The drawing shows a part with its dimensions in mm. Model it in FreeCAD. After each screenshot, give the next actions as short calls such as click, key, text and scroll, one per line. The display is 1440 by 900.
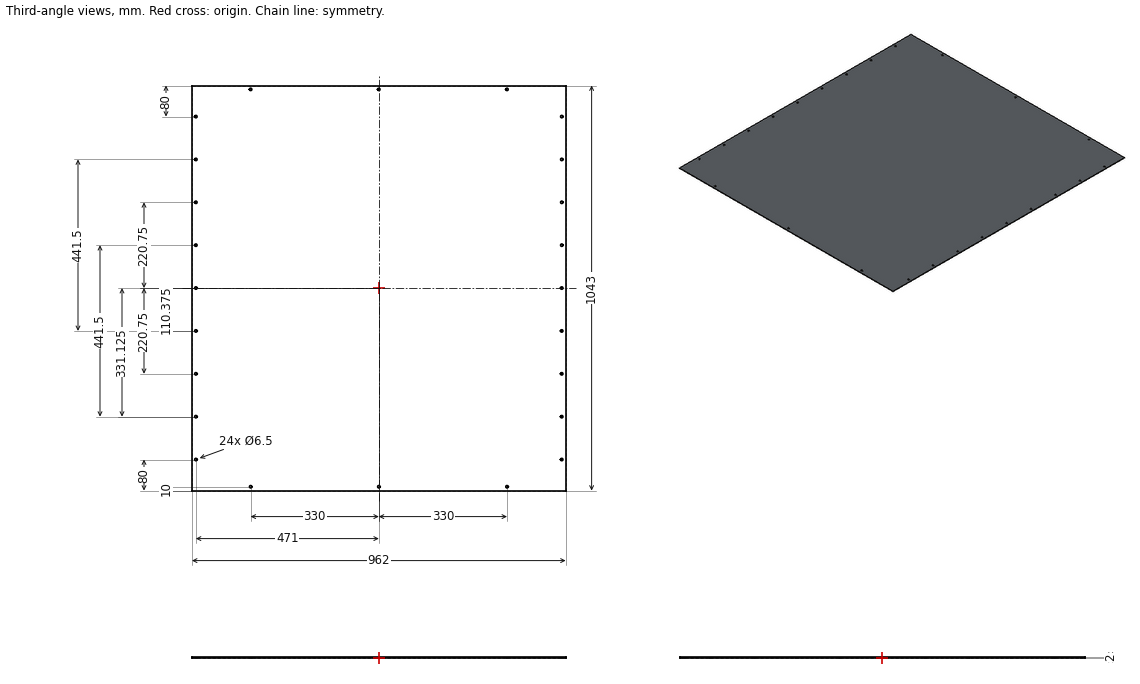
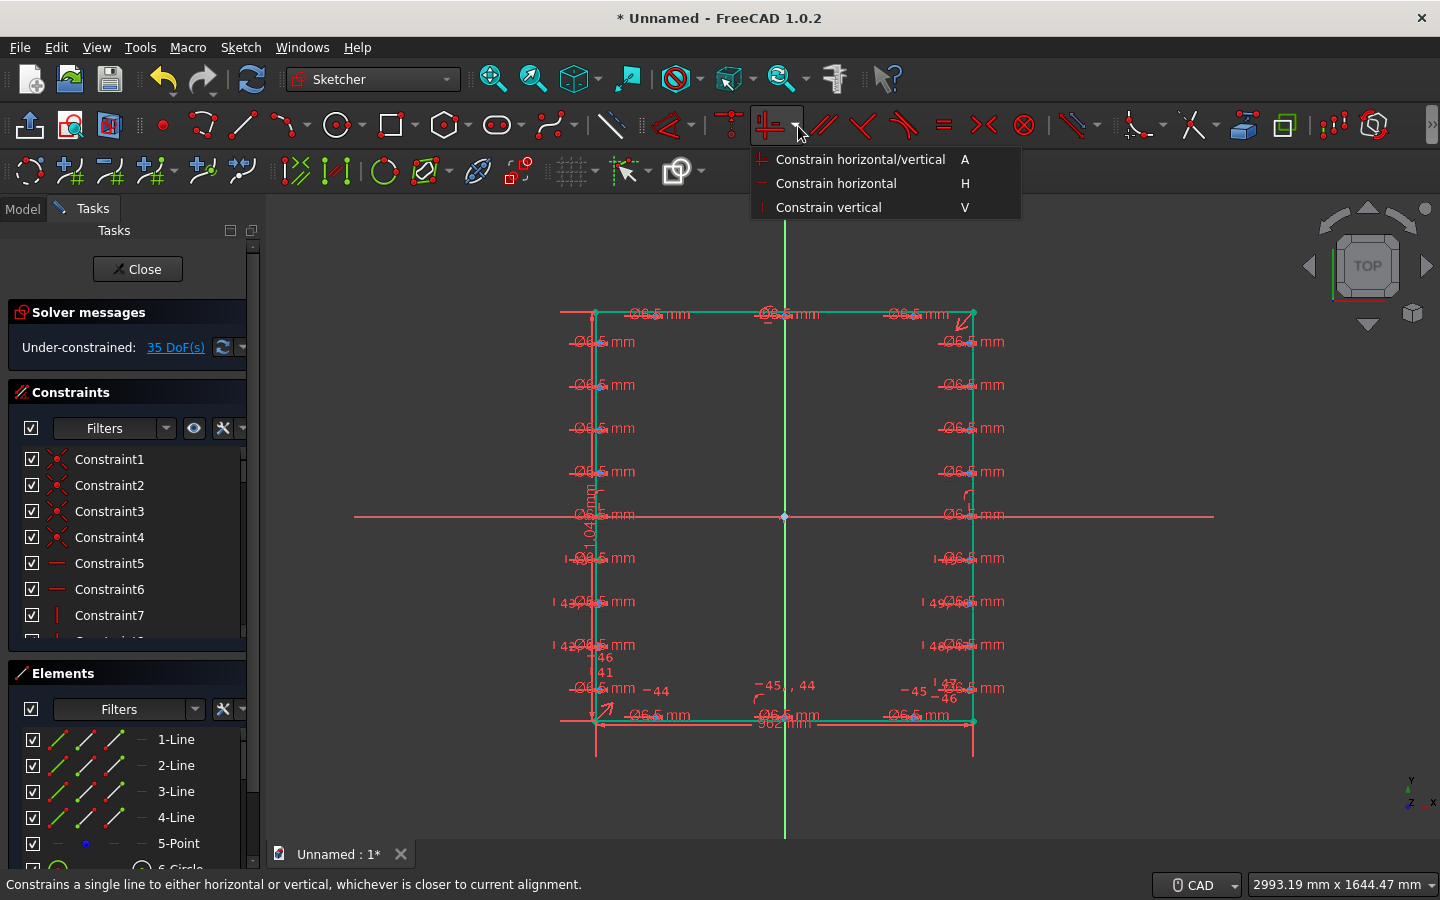
click(886, 207)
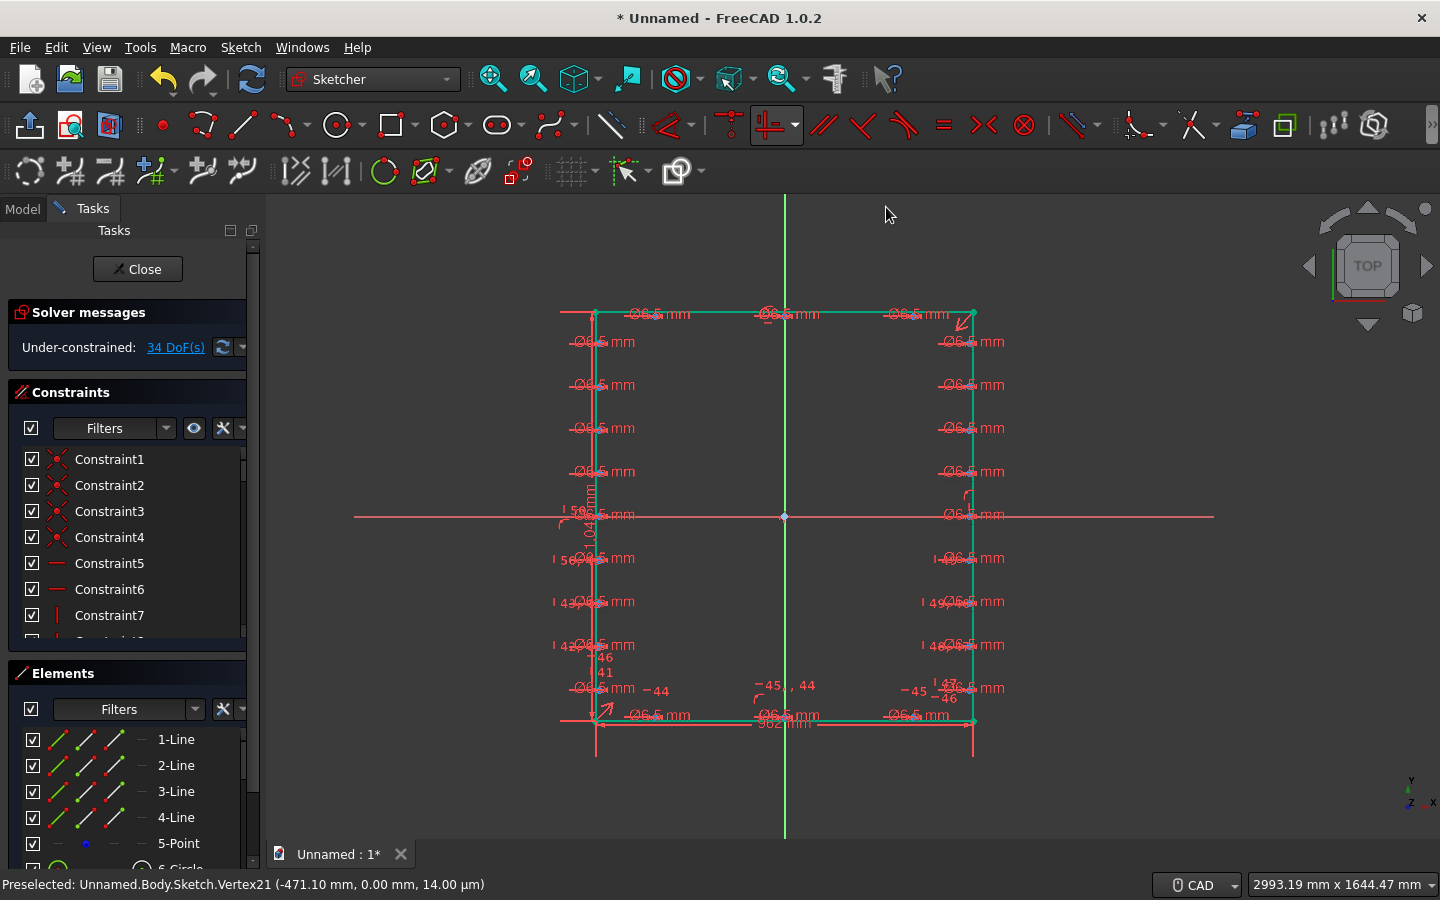
click(600, 517)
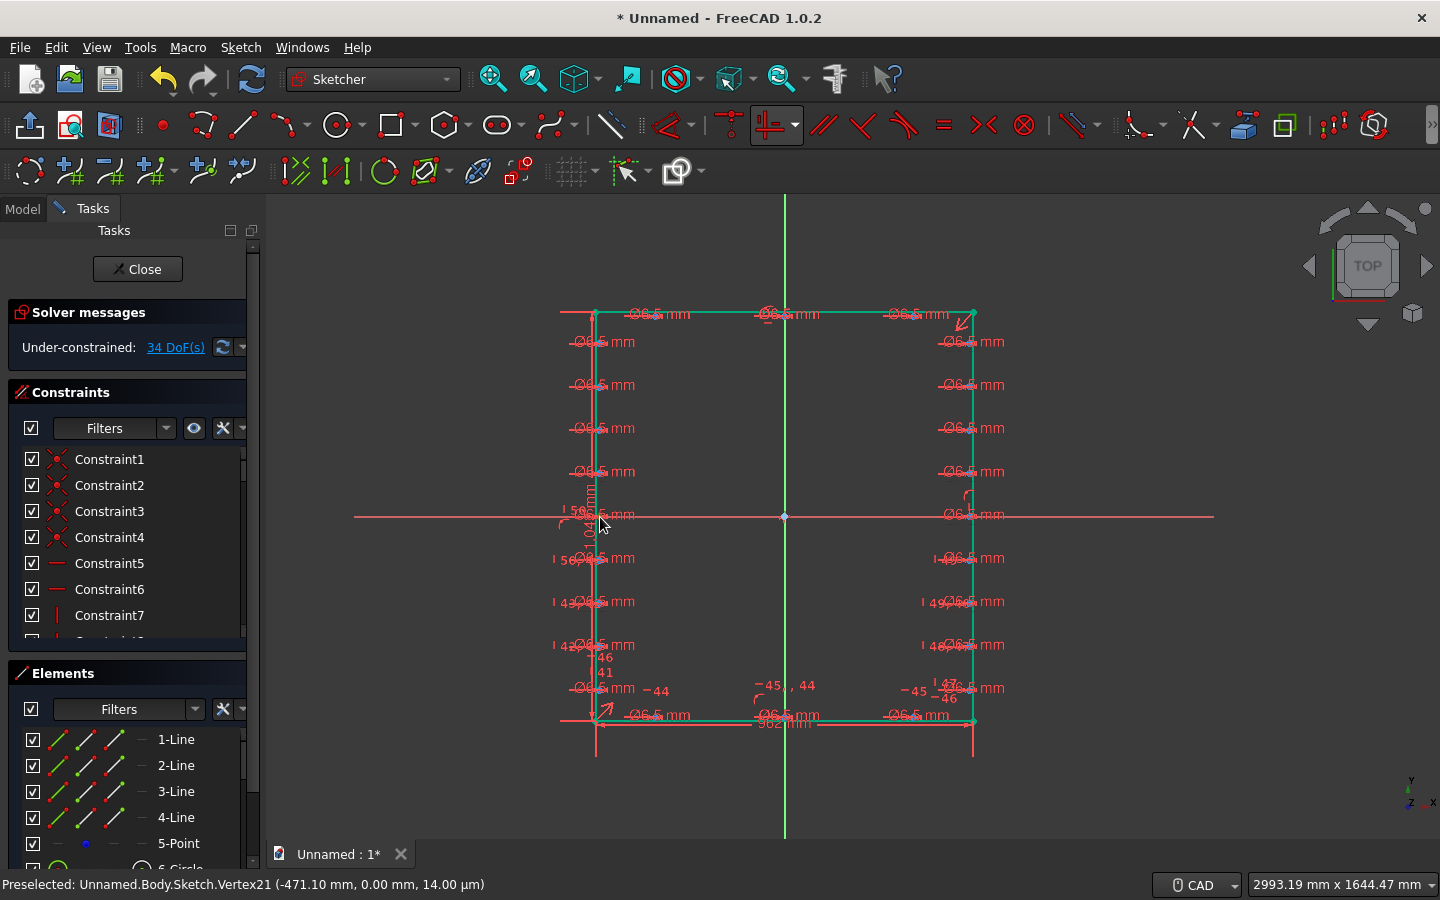
click(600, 474)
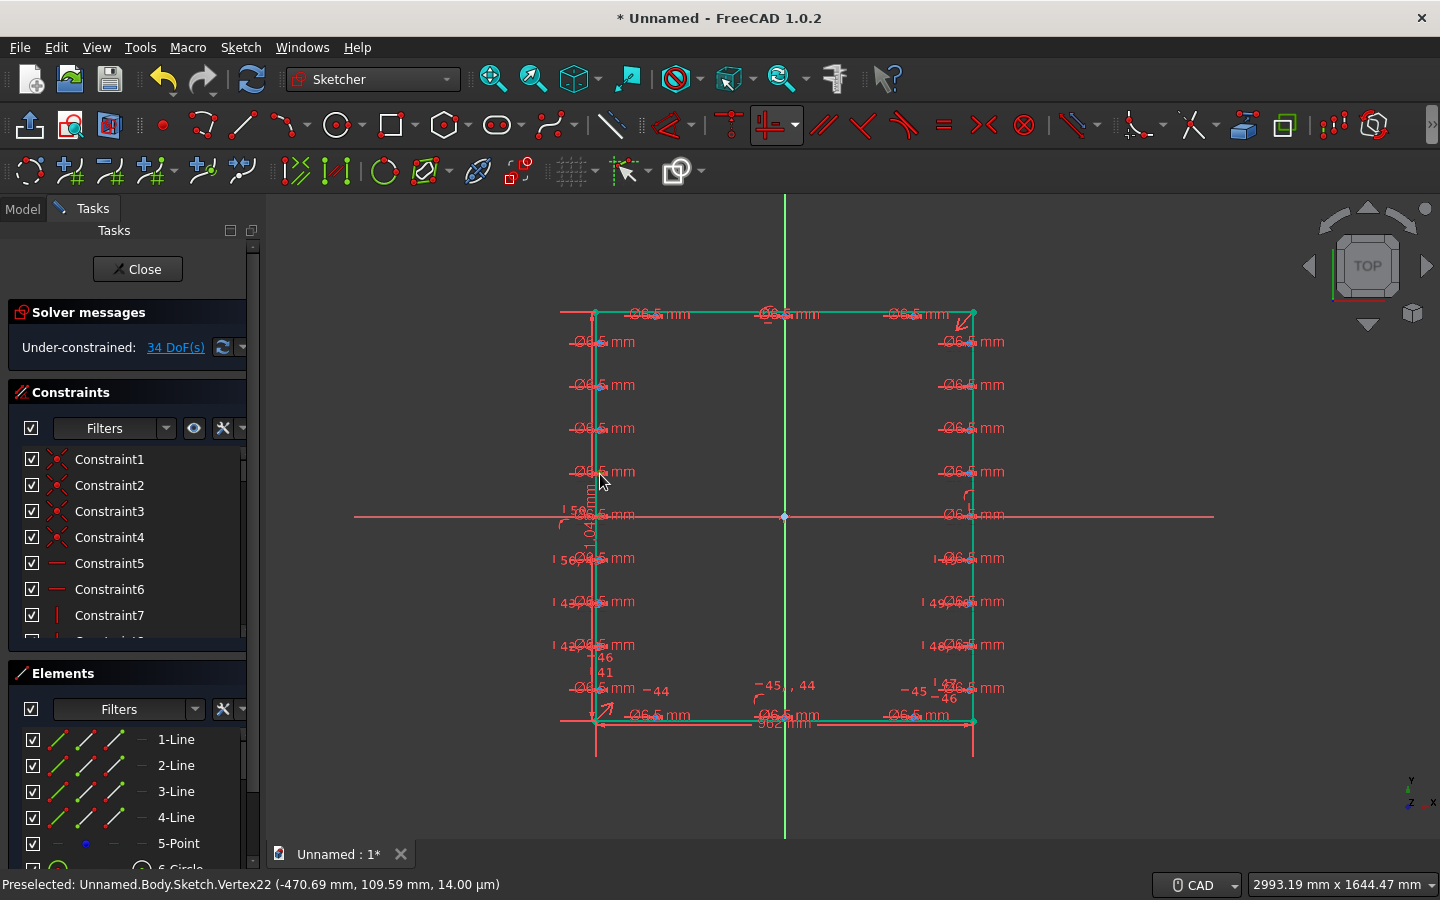
click(798, 126)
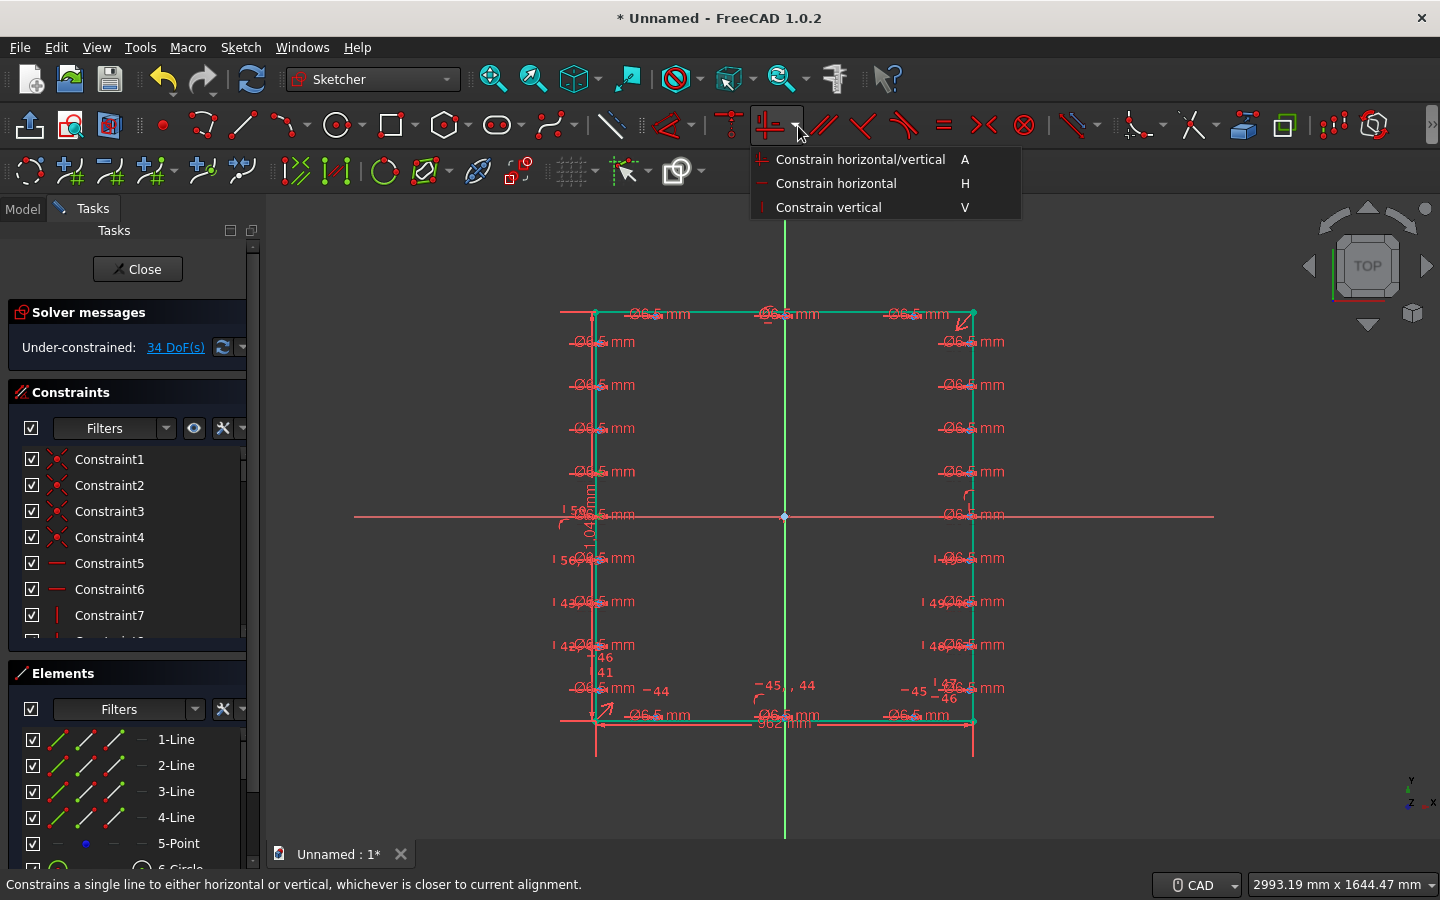
click(886, 207)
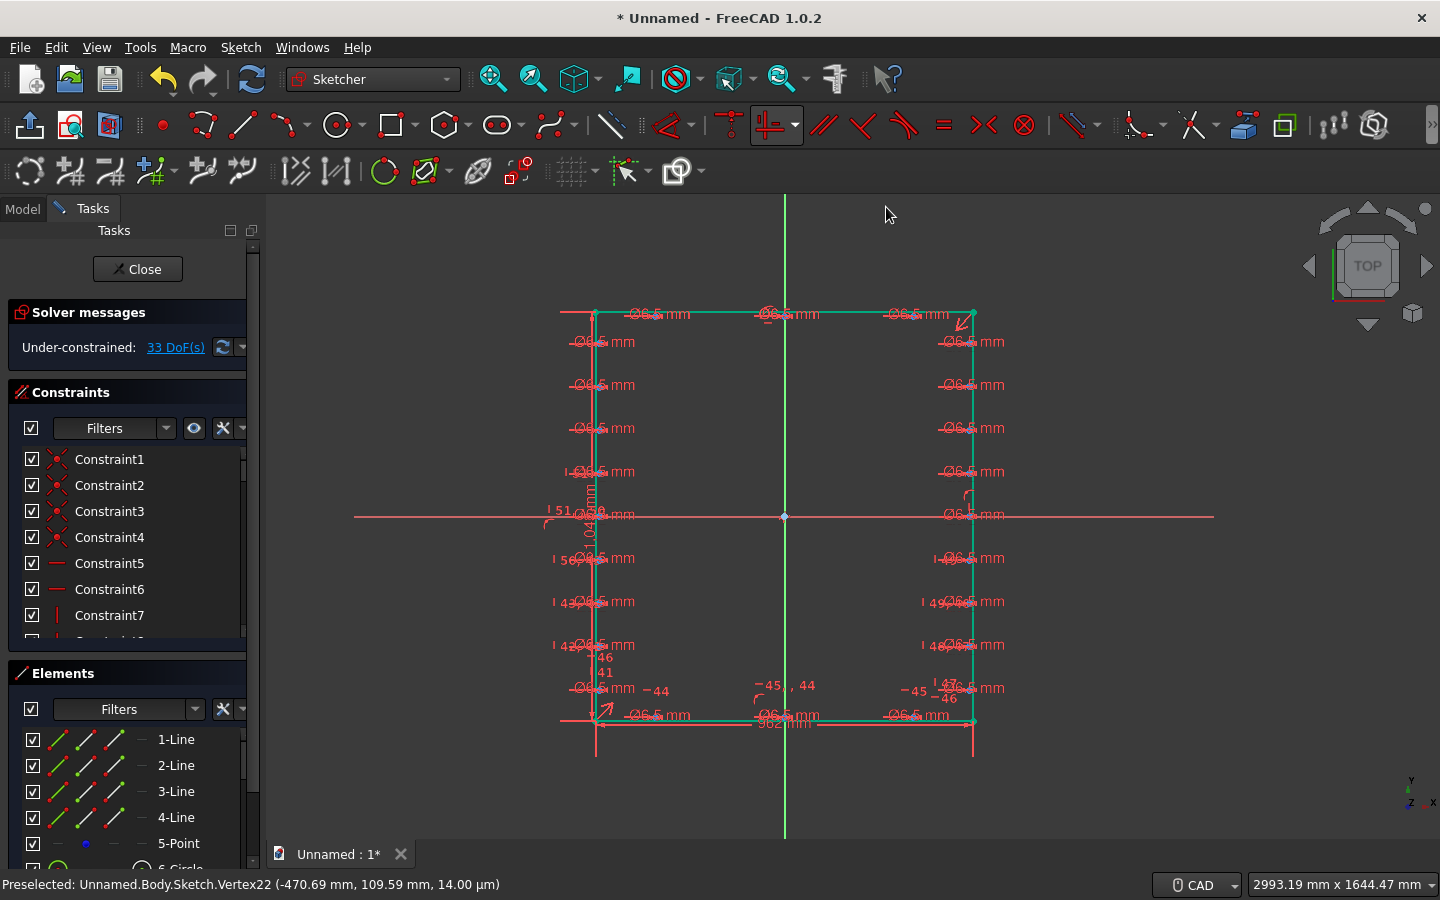
click(600, 474)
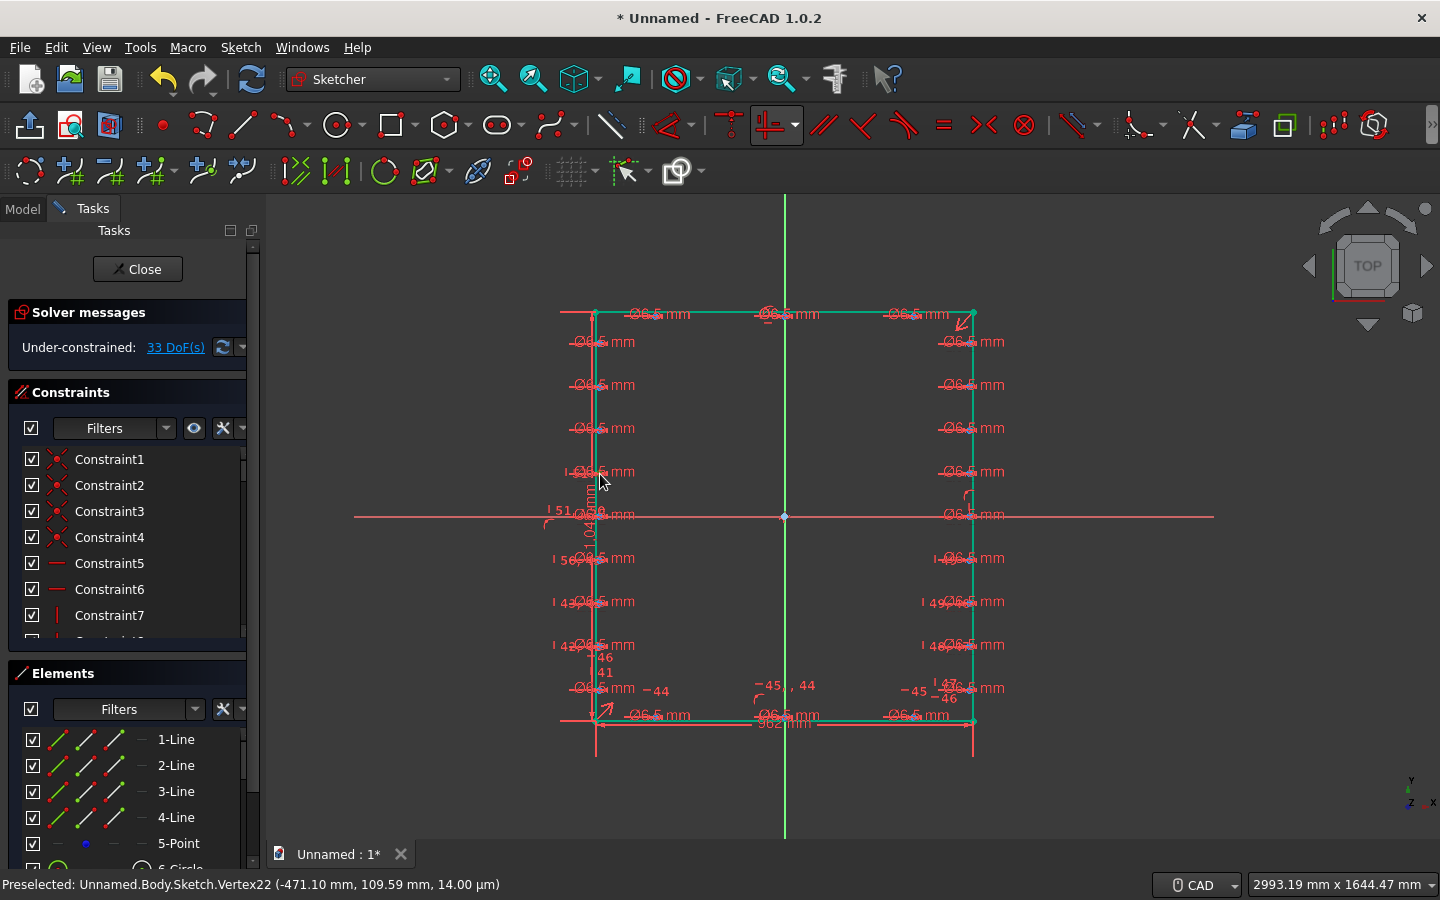
click(600, 430)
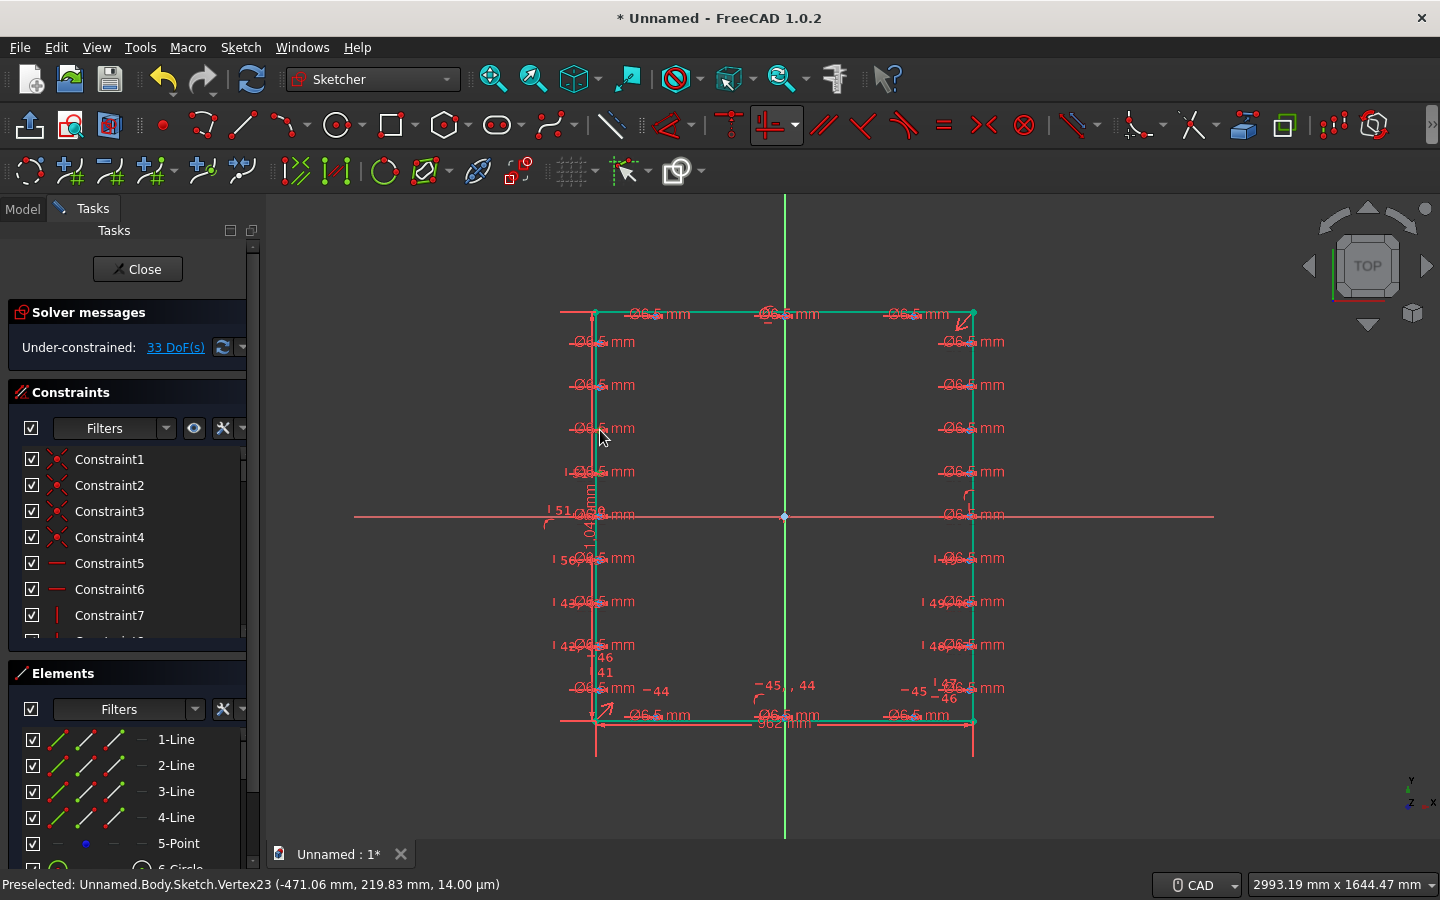
click(798, 126)